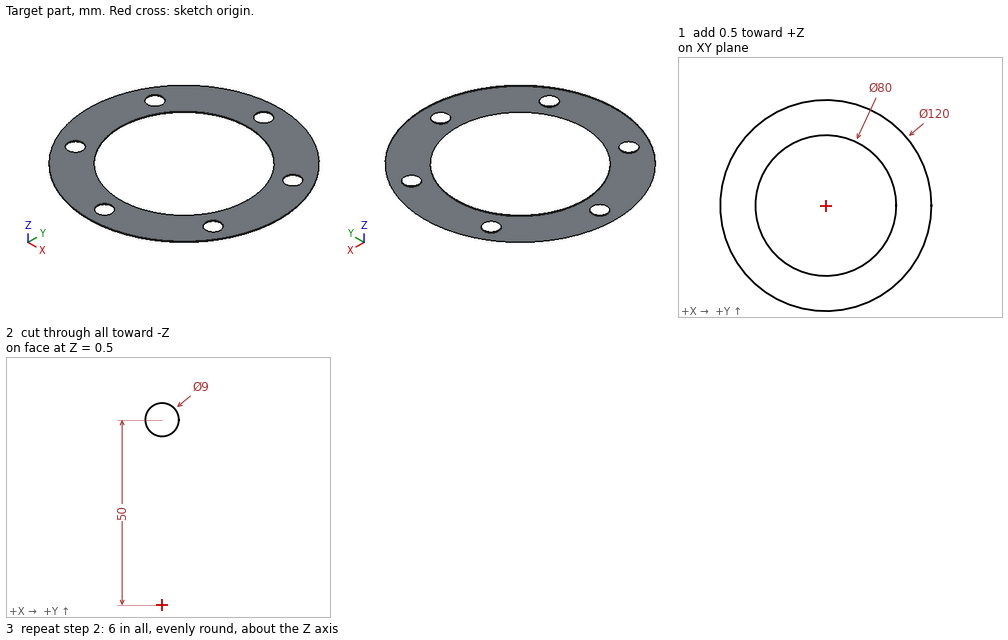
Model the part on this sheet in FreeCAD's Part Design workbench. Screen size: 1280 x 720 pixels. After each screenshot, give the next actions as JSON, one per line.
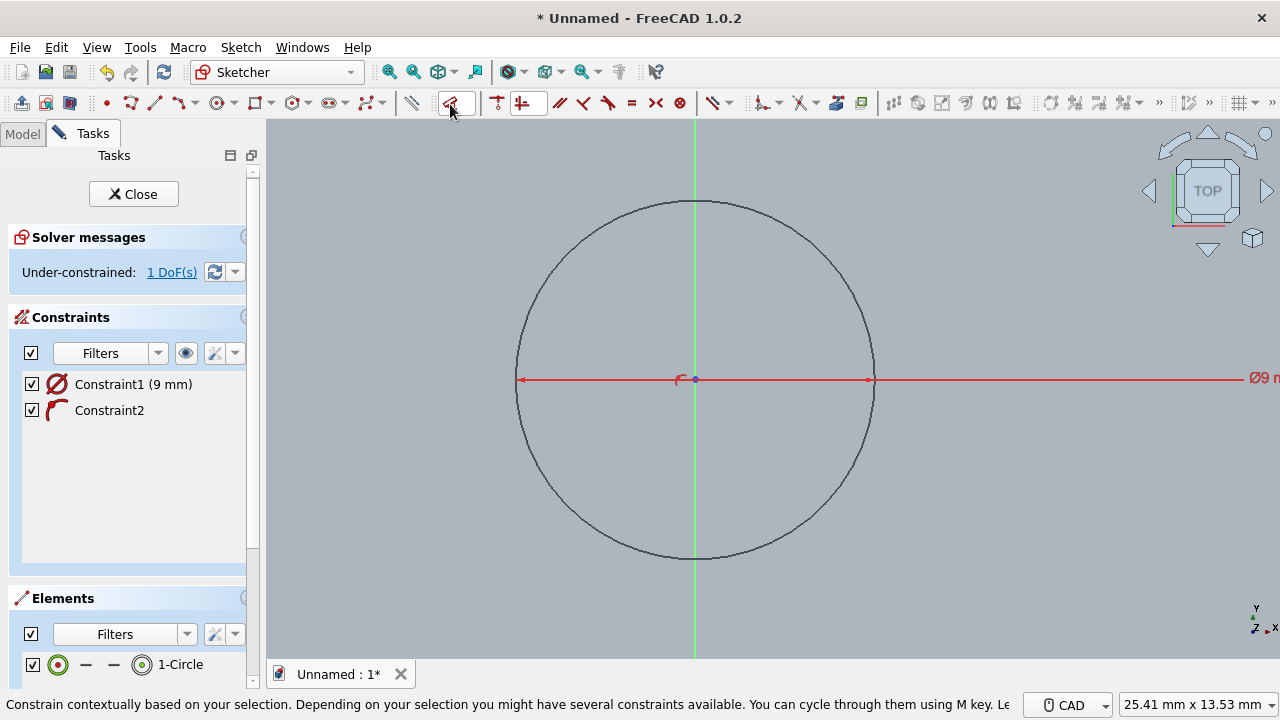
{"action": "left_click", "coordinate": [695, 380]}
{"action": "left_click", "coordinate": [729, 505]}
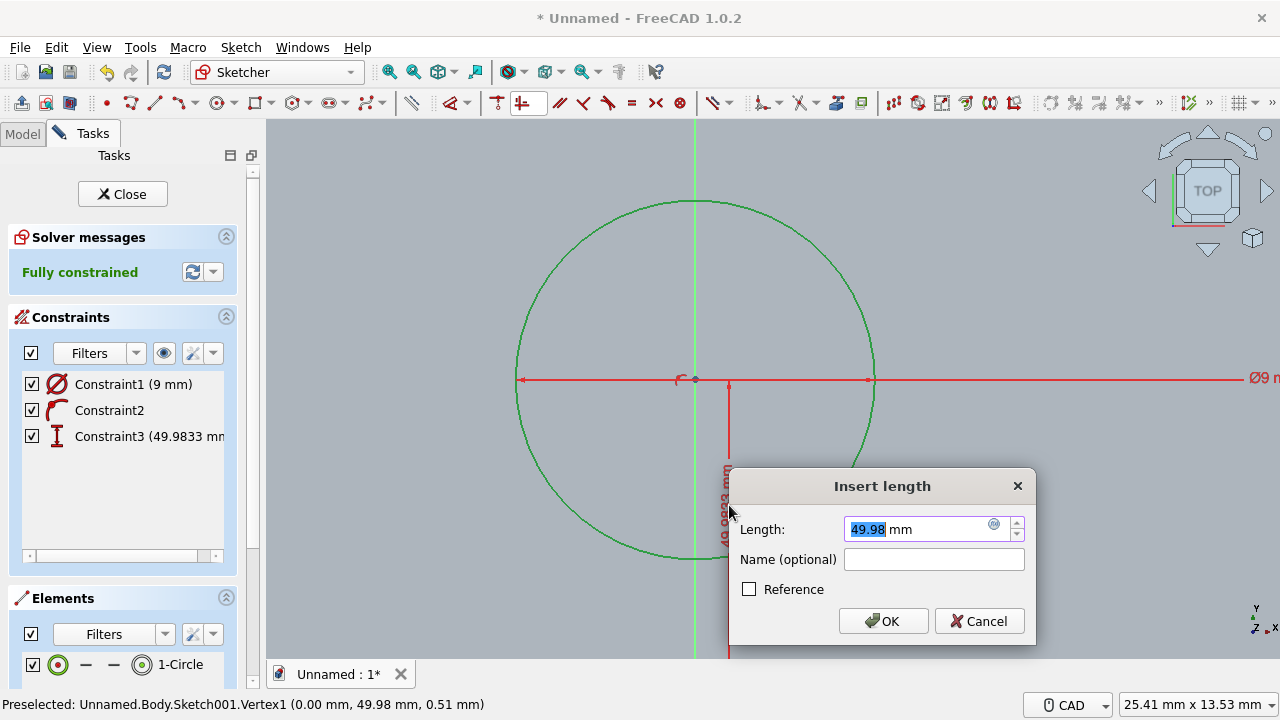
{"action": "type", "text": "50"}
{"action": "key", "text": "Return"}
{"action": "key", "text": "Escape"}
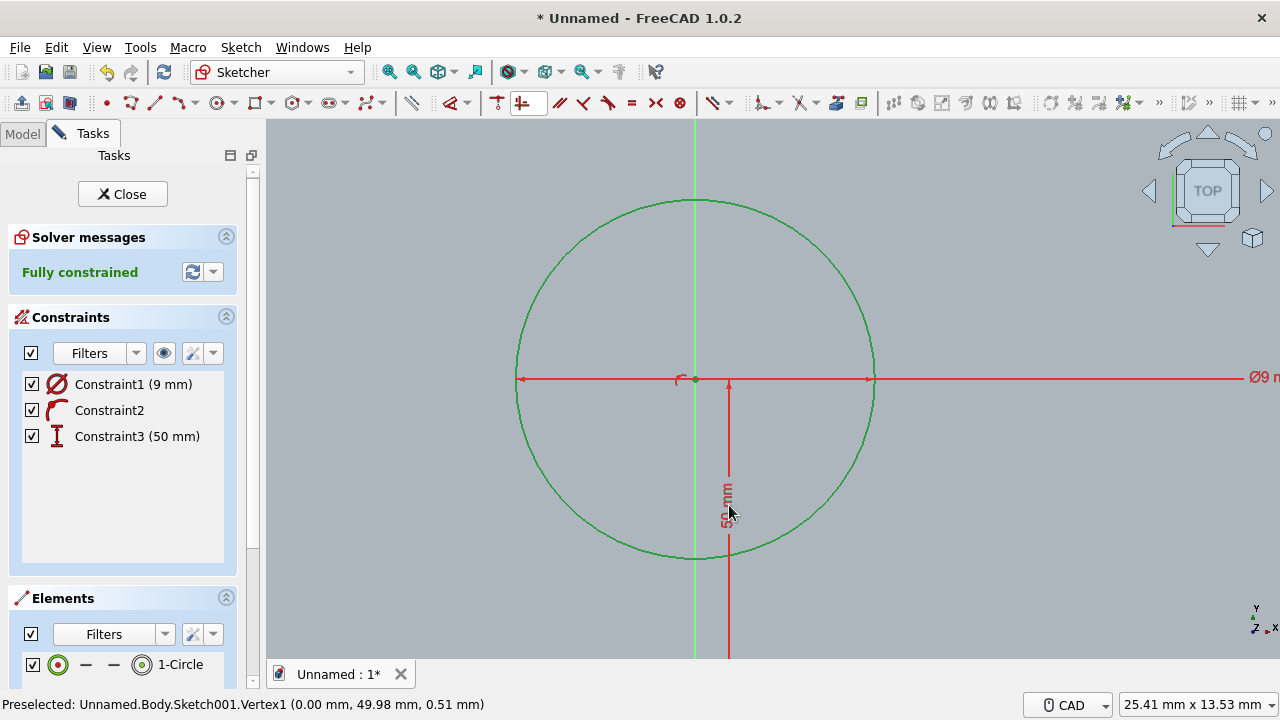
{"action": "left_click", "coordinate": [123, 194]}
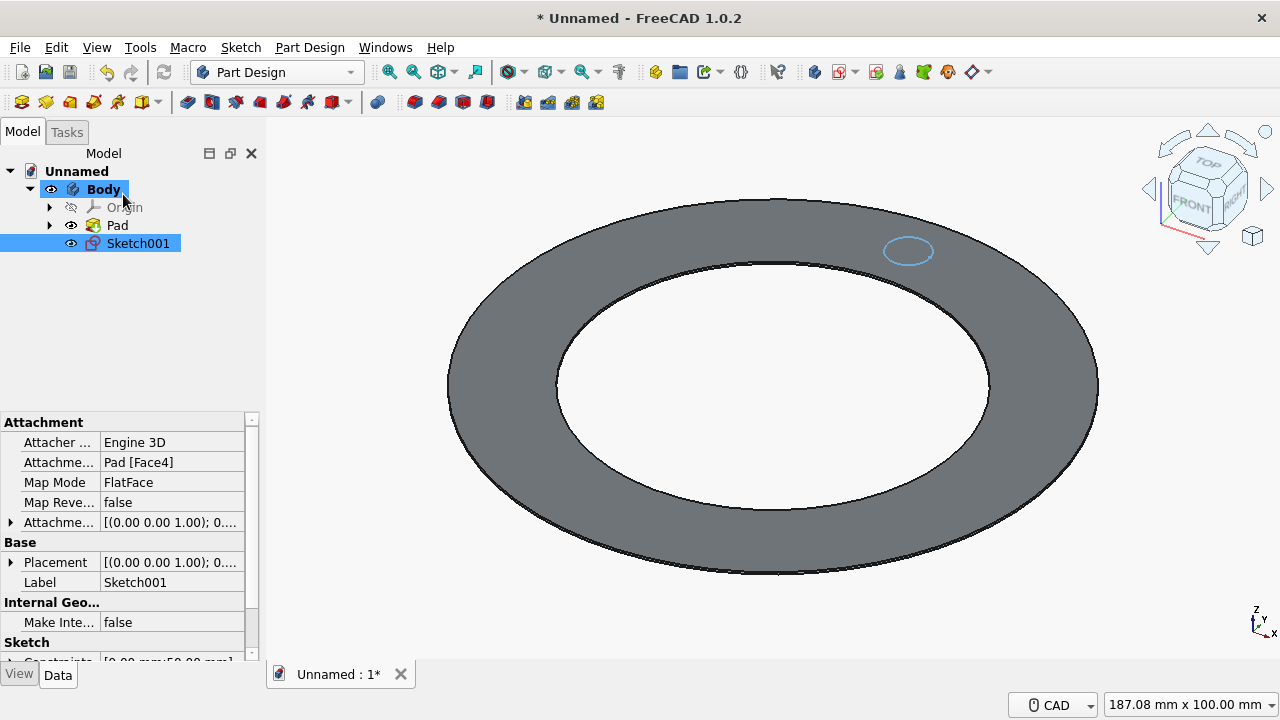
{"action": "left_click", "coordinate": [188, 102]}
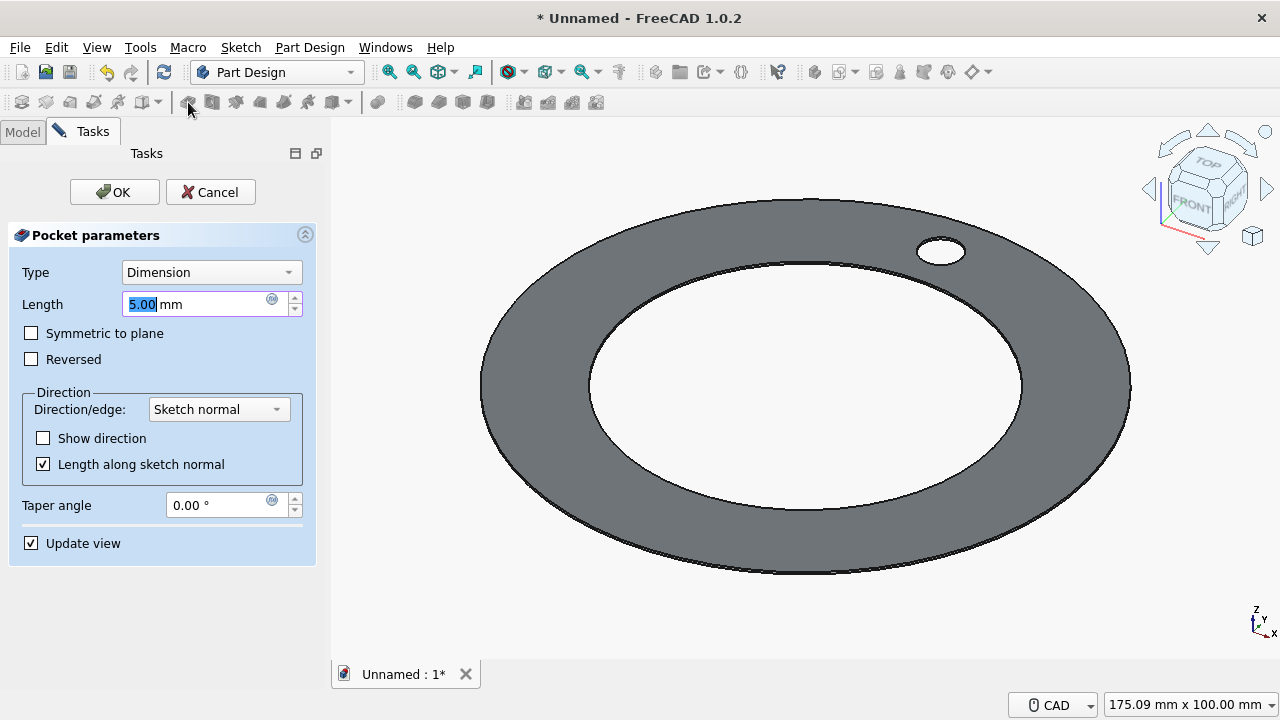
{"action": "left_click", "coordinate": [212, 272]}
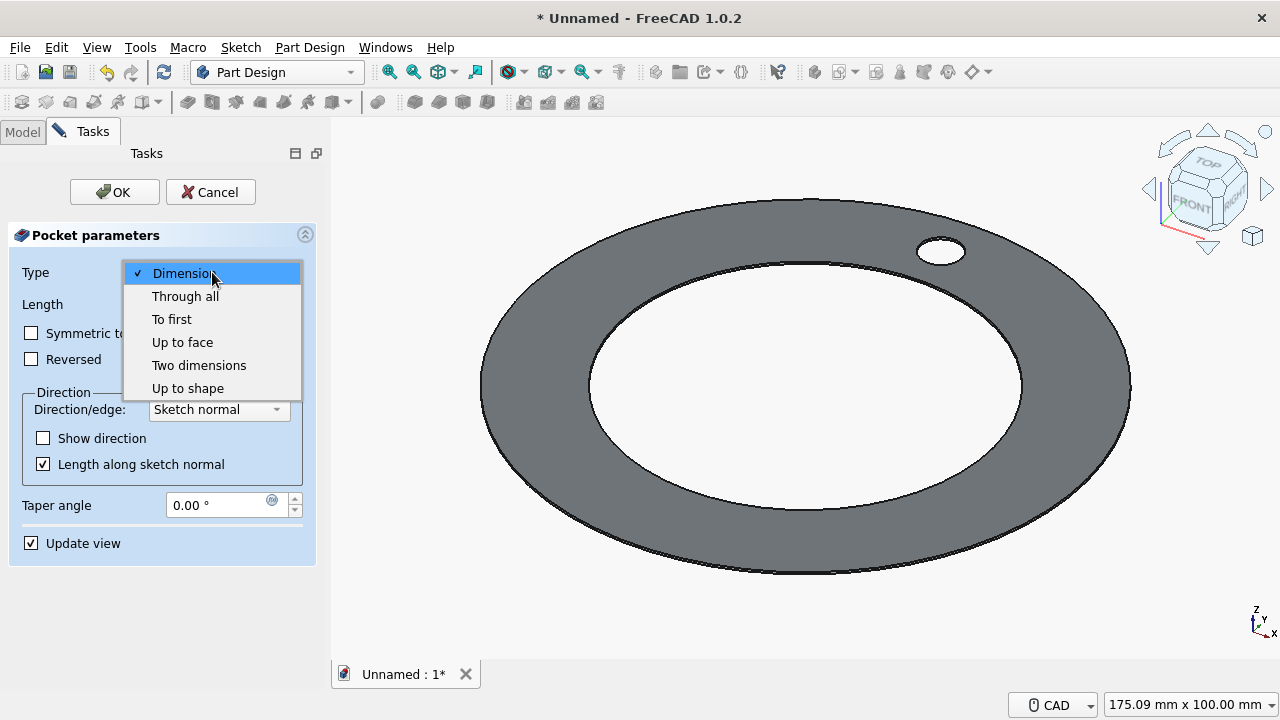
{"action": "left_click", "coordinate": [212, 296]}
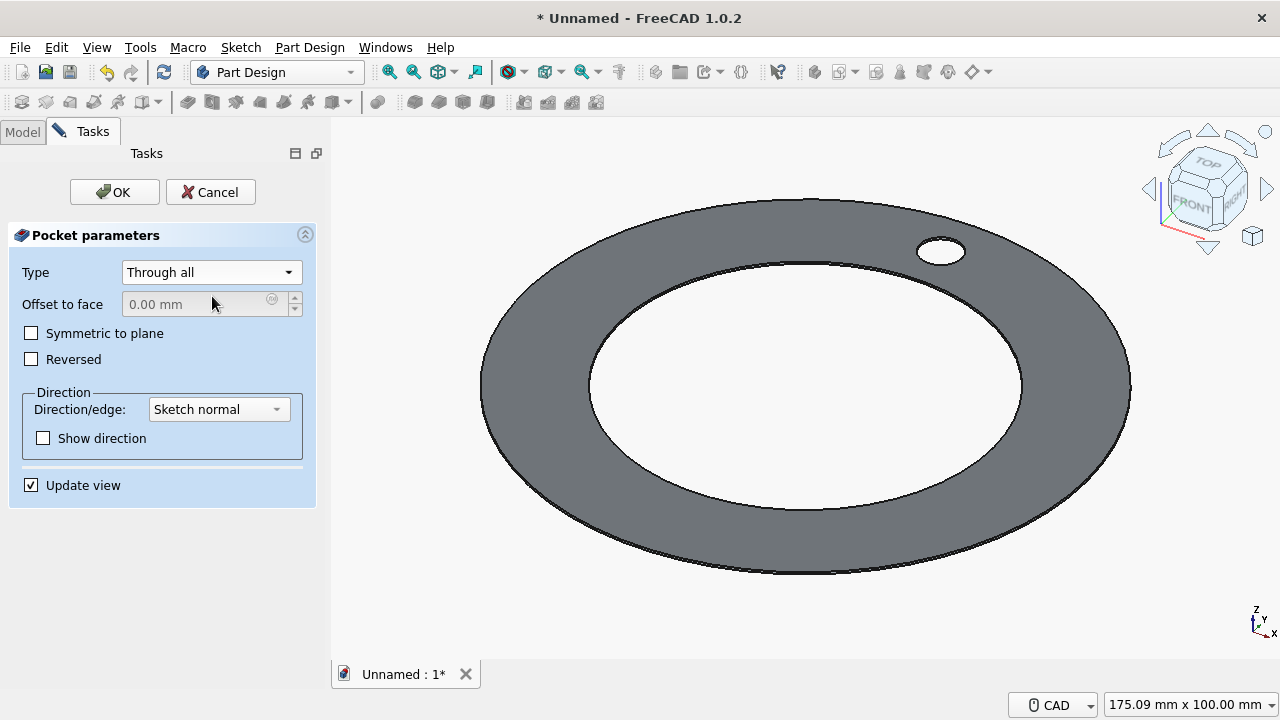
{"action": "left_click", "coordinate": [115, 192]}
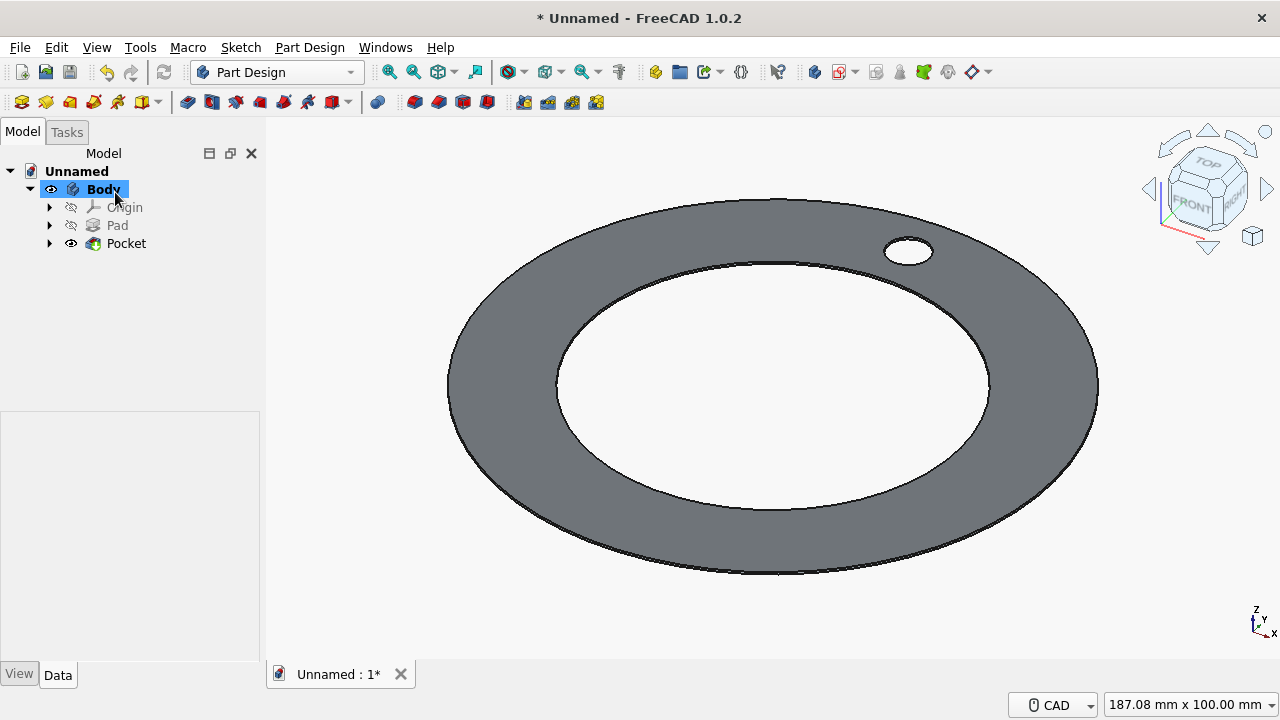
{"action": "left_click", "coordinate": [116, 243]}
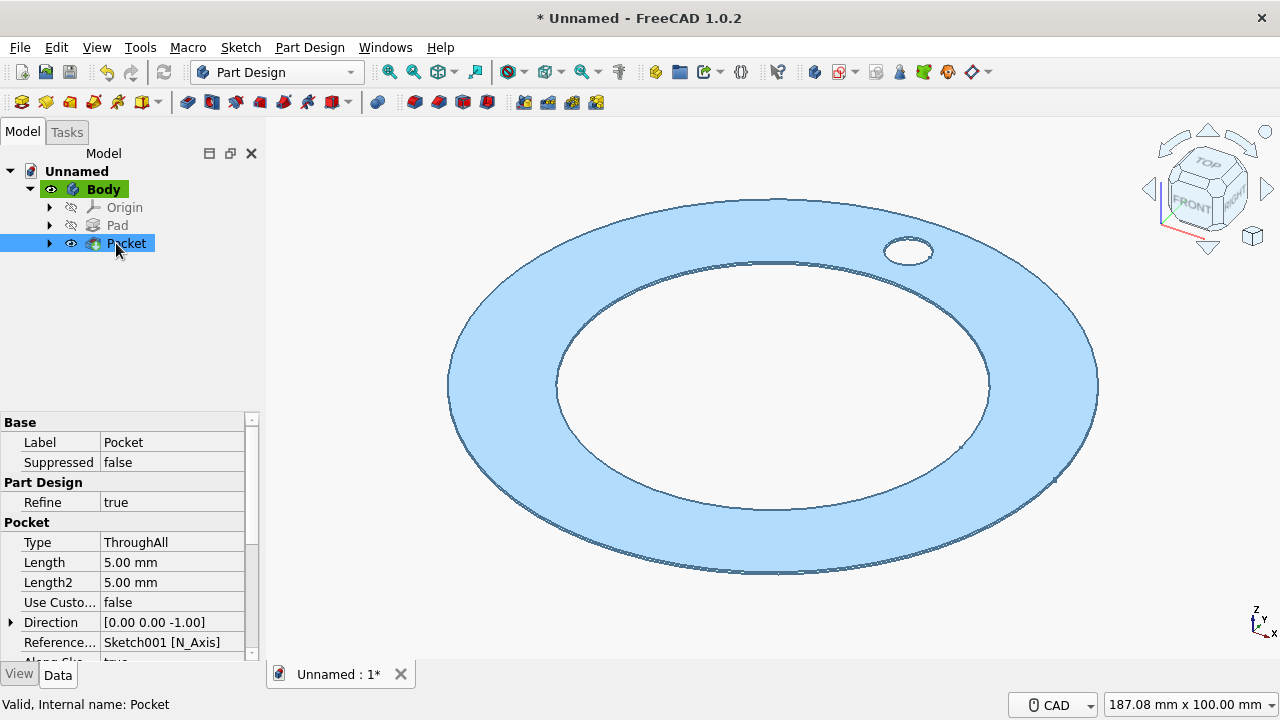
{"action": "left_click", "coordinate": [572, 102]}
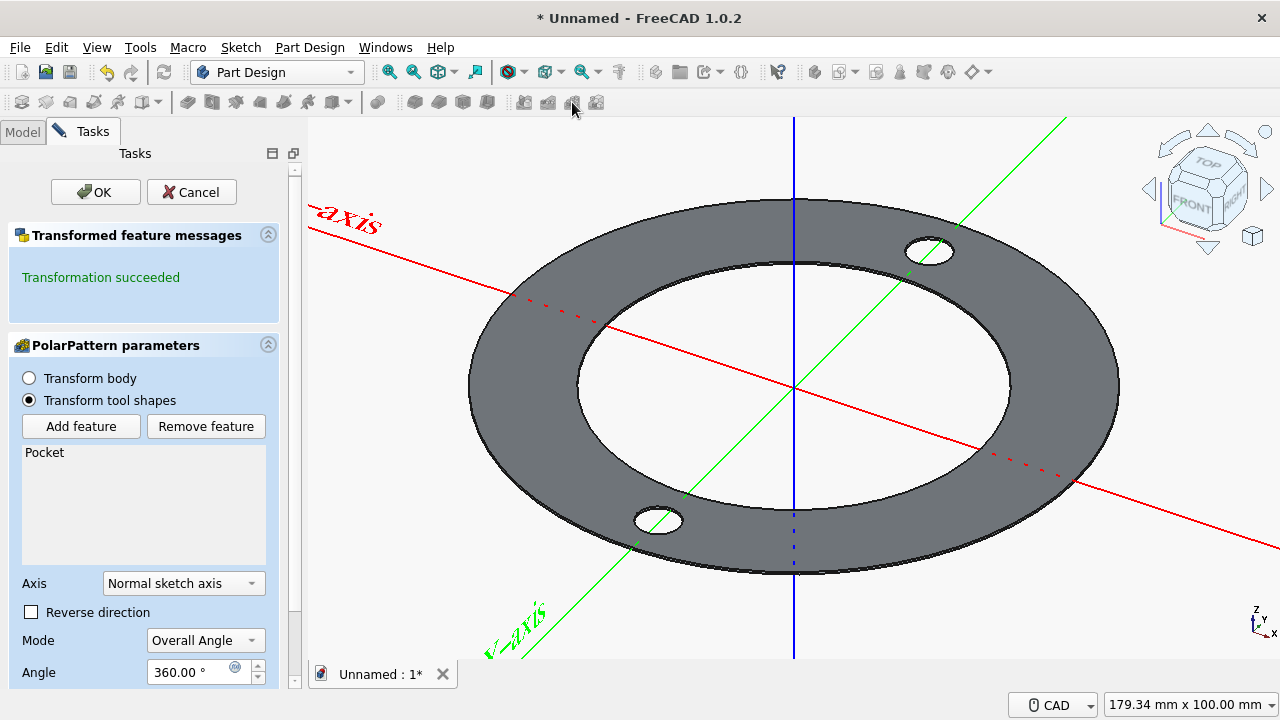
{"action": "left_click", "coordinate": [184, 584]}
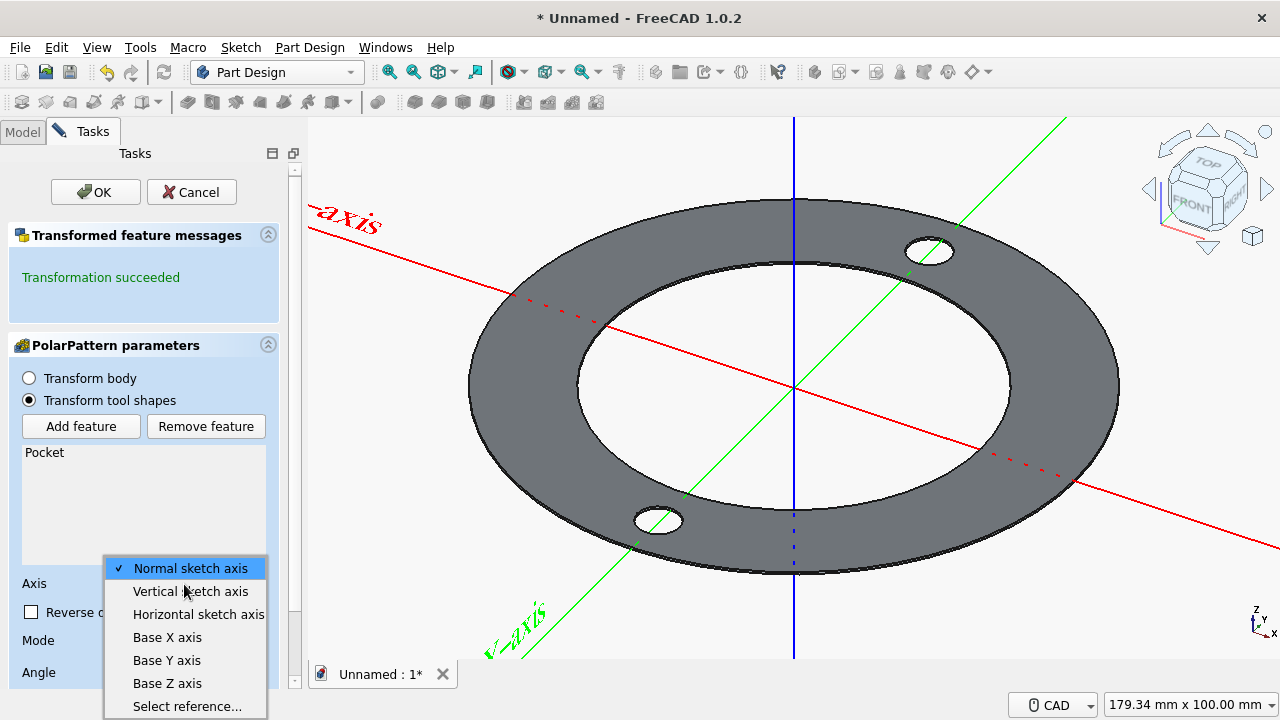
{"action": "left_click", "coordinate": [184, 684]}